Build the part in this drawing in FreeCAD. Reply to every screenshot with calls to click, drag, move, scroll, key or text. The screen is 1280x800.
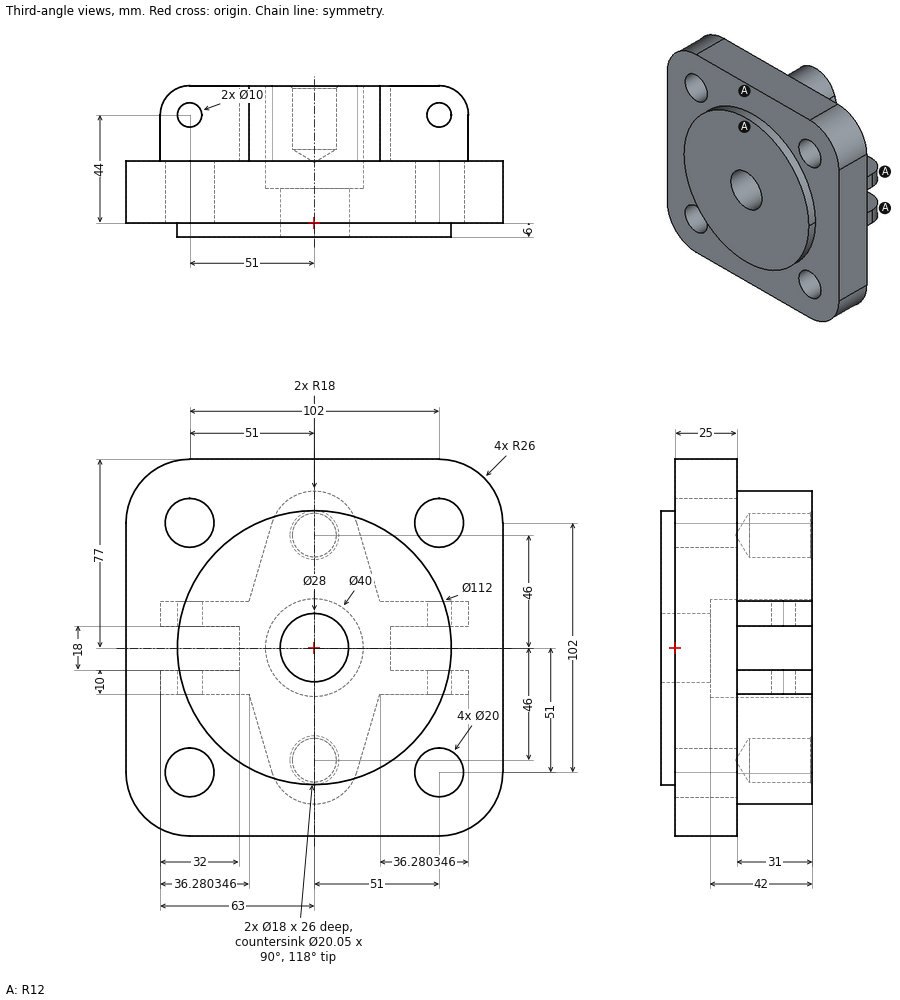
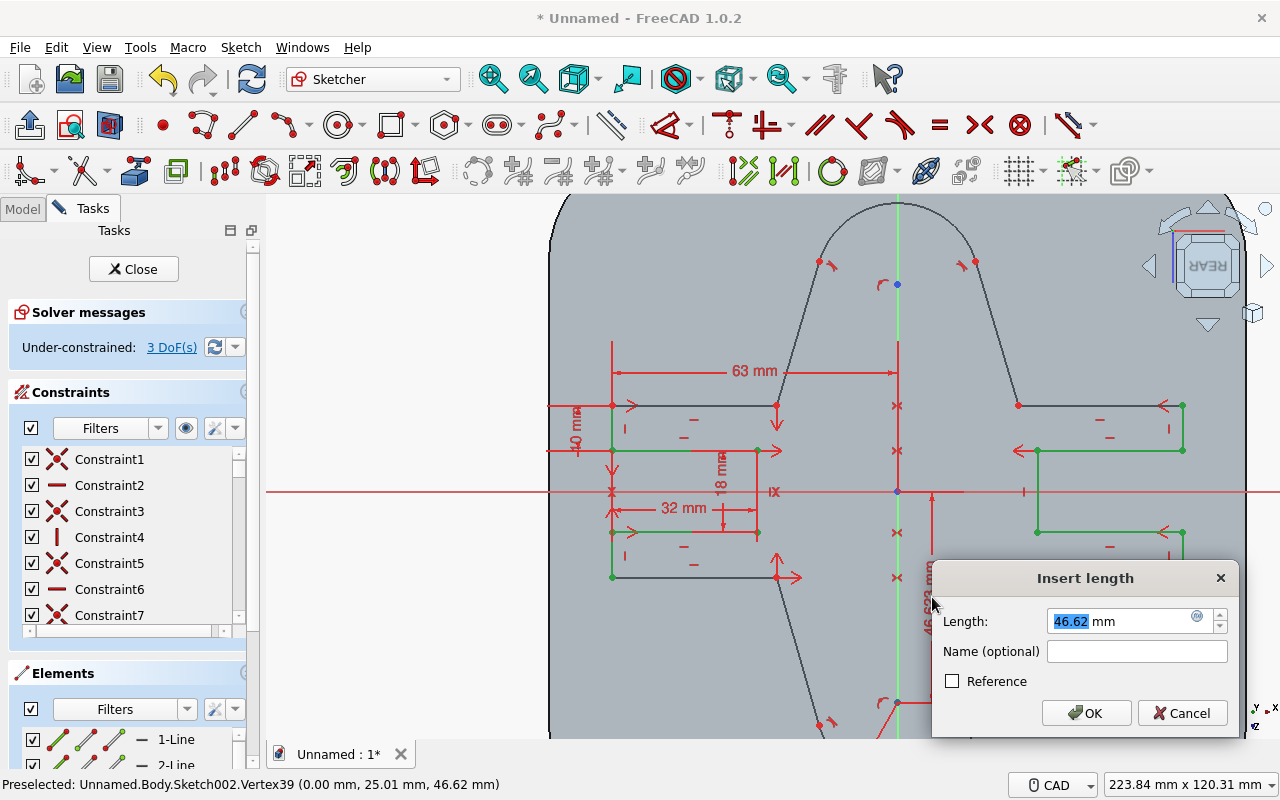
text(46)
key(Return)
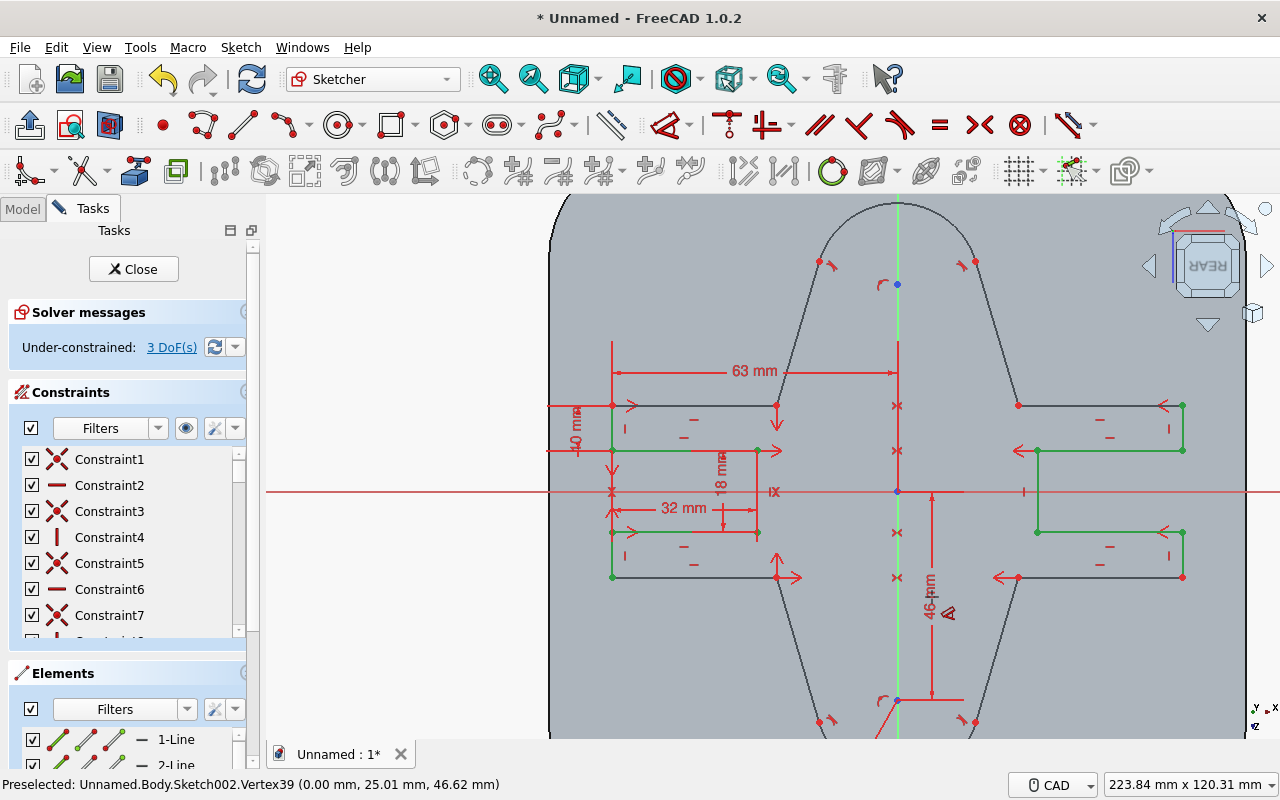
click(898, 285)
click(932, 388)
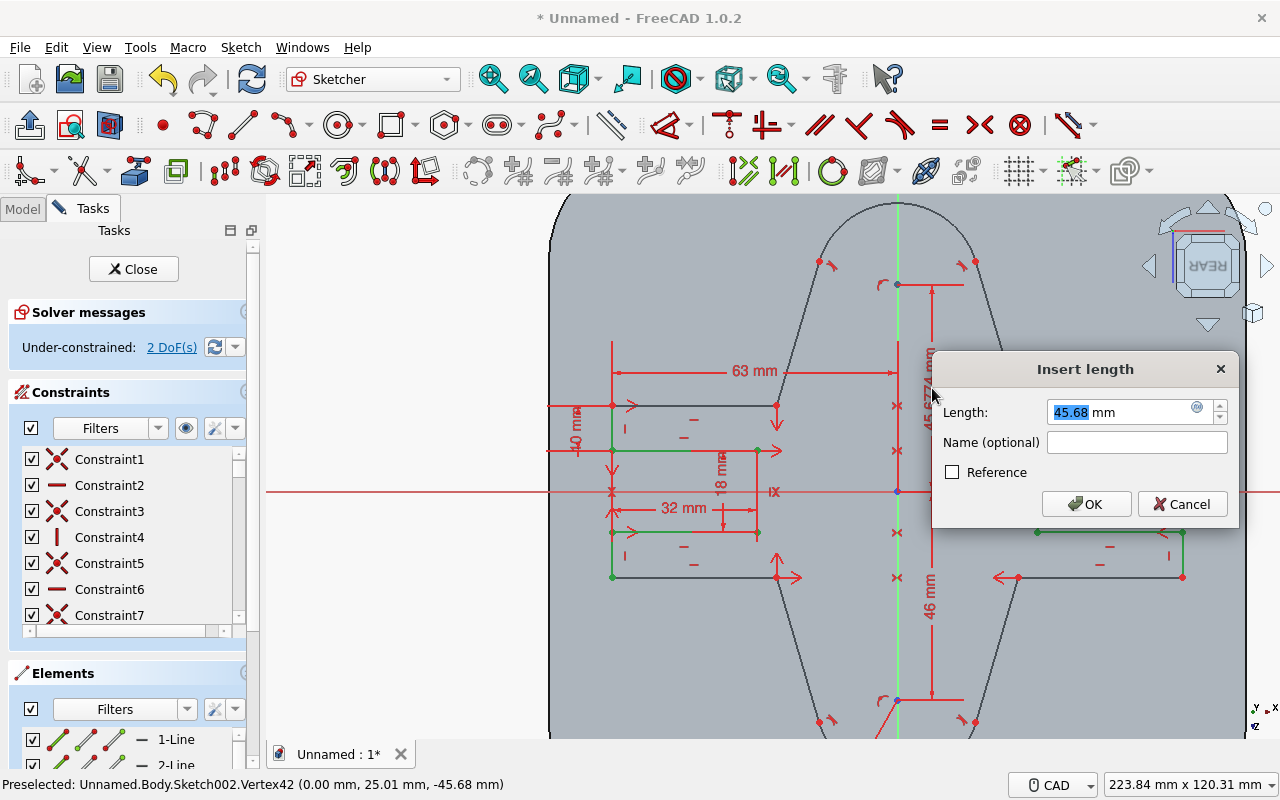
text(46)
key(Return)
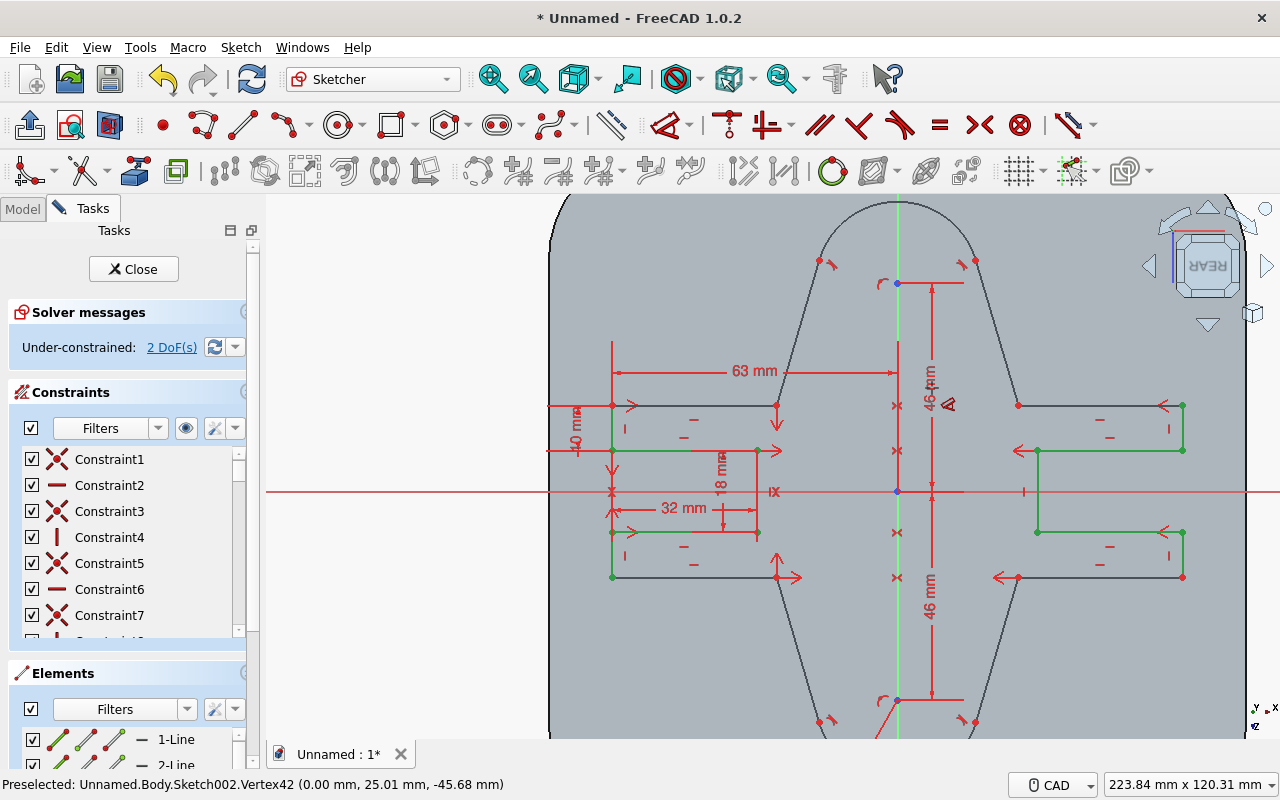
click(727, 406)
click(657, 372)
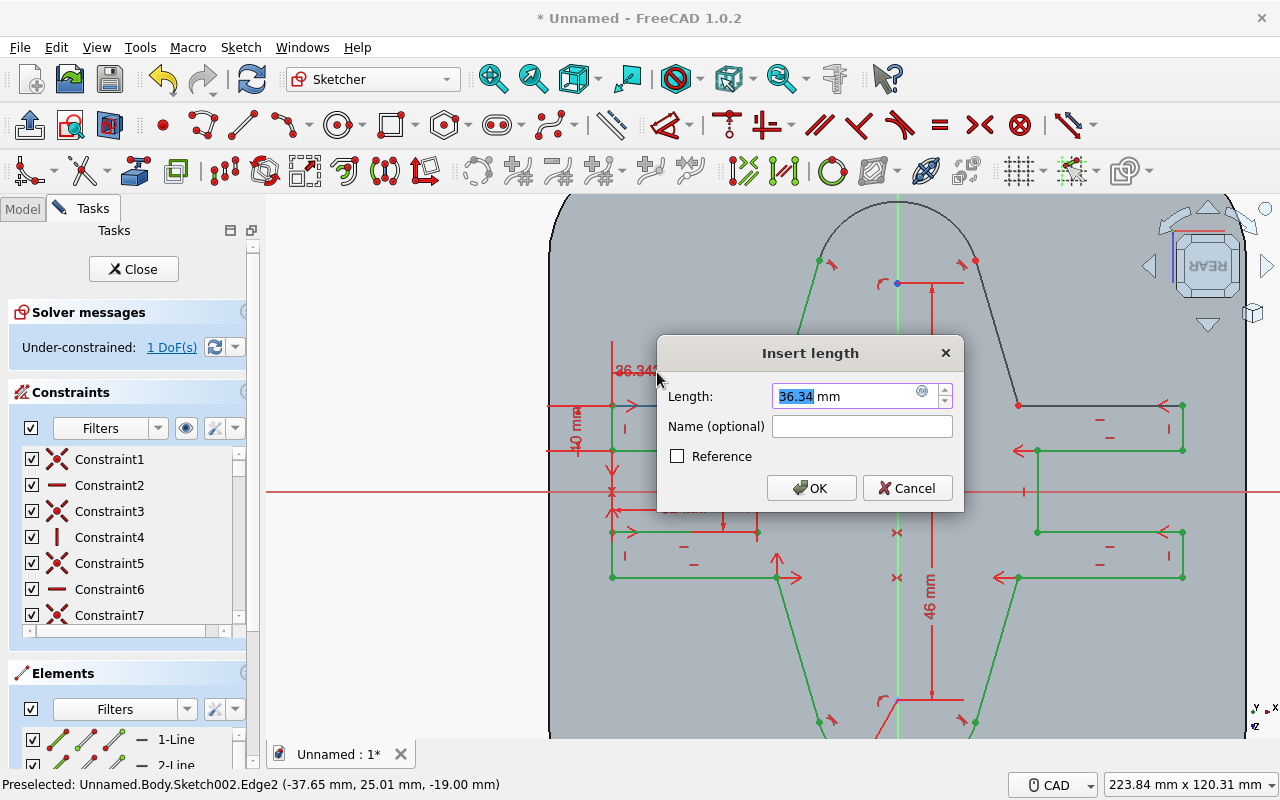
text(36.280346)
key(Return)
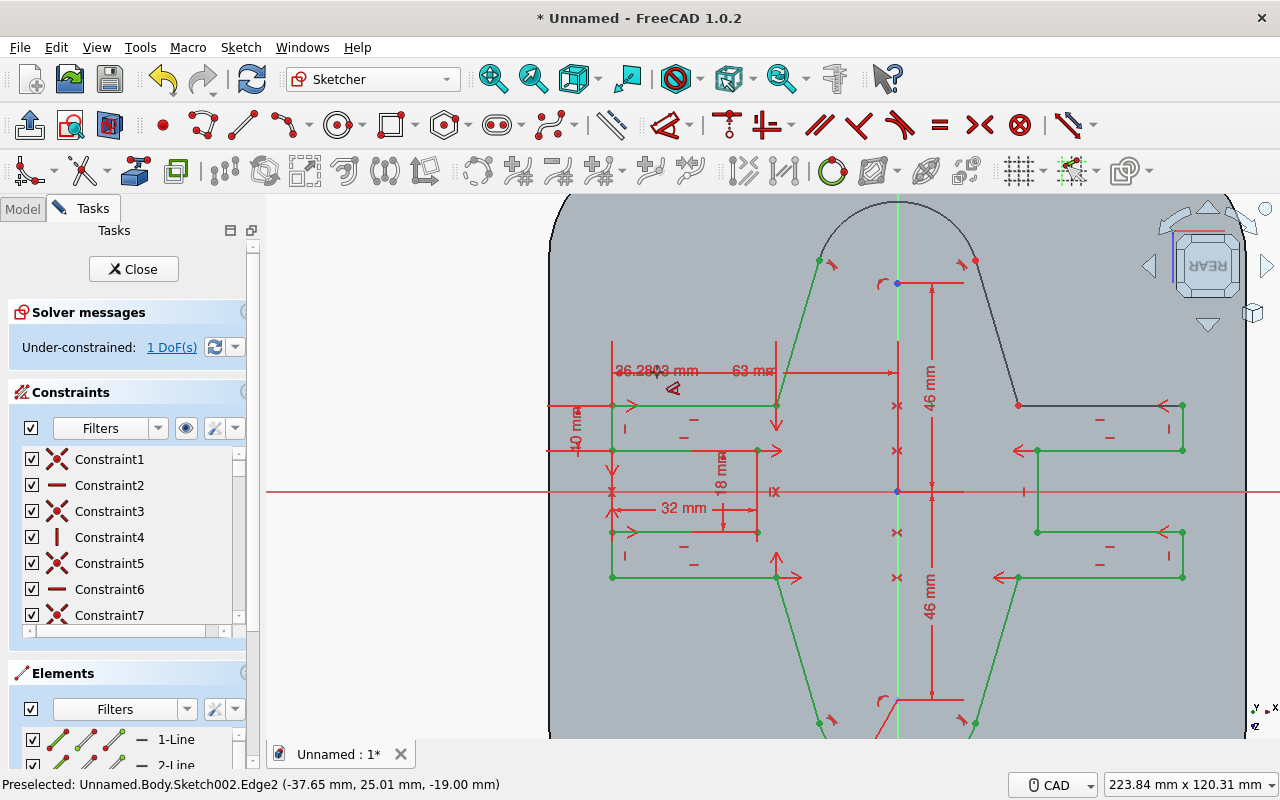
click(1068, 406)
click(1067, 372)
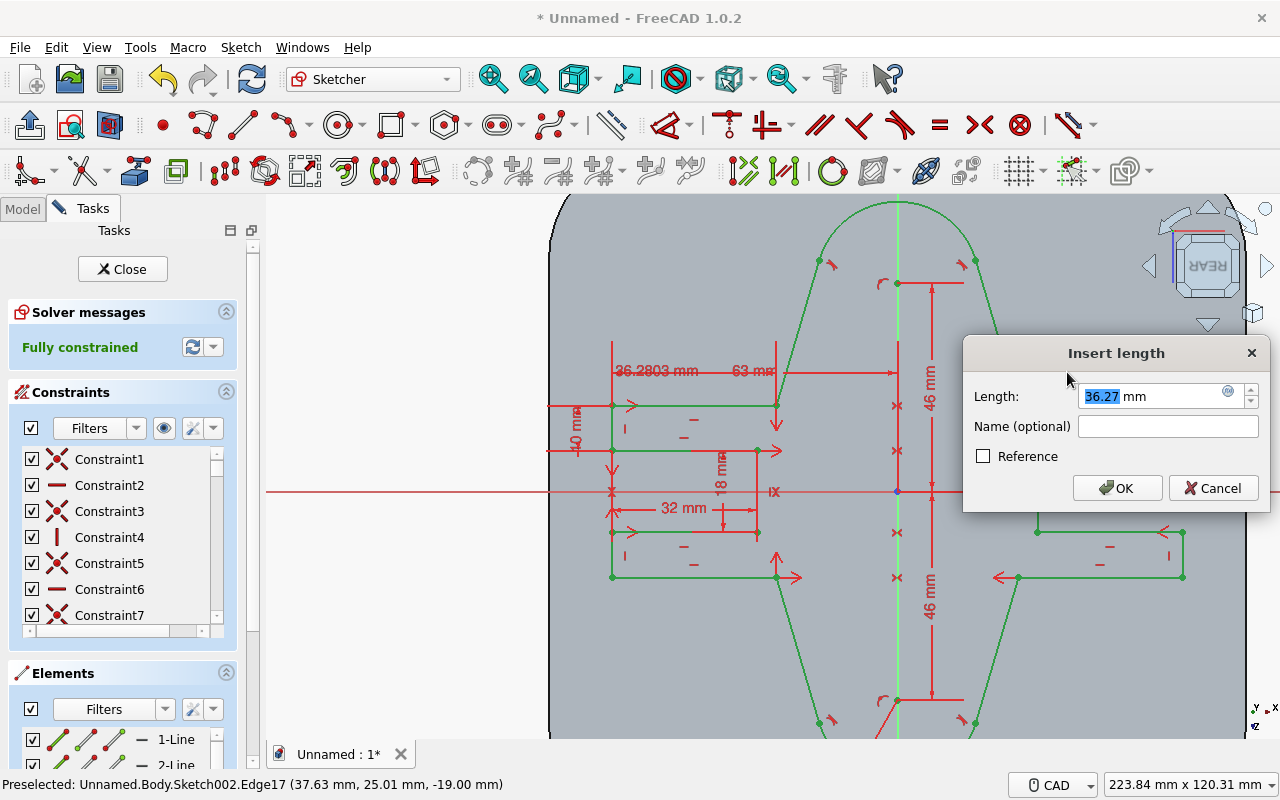
text(36.280346)
key(Return)
key(Escape)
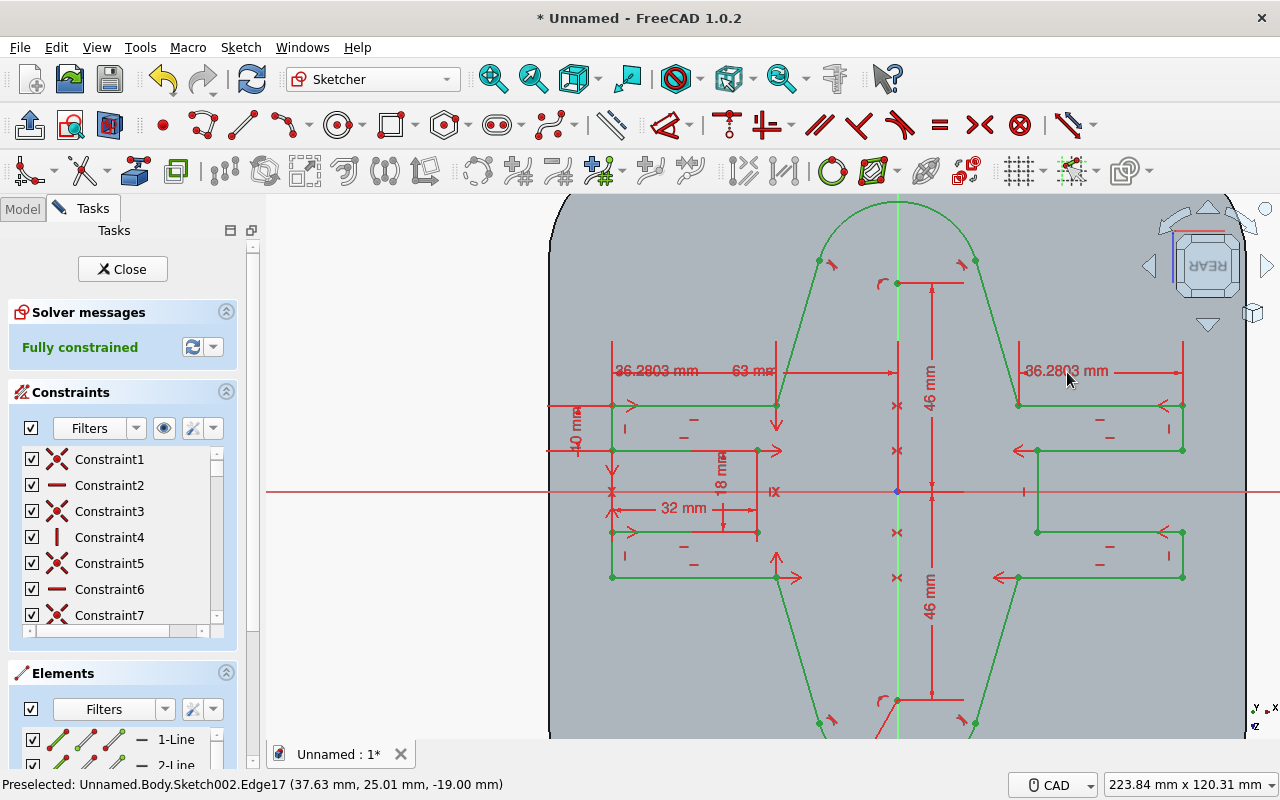
click(123, 269)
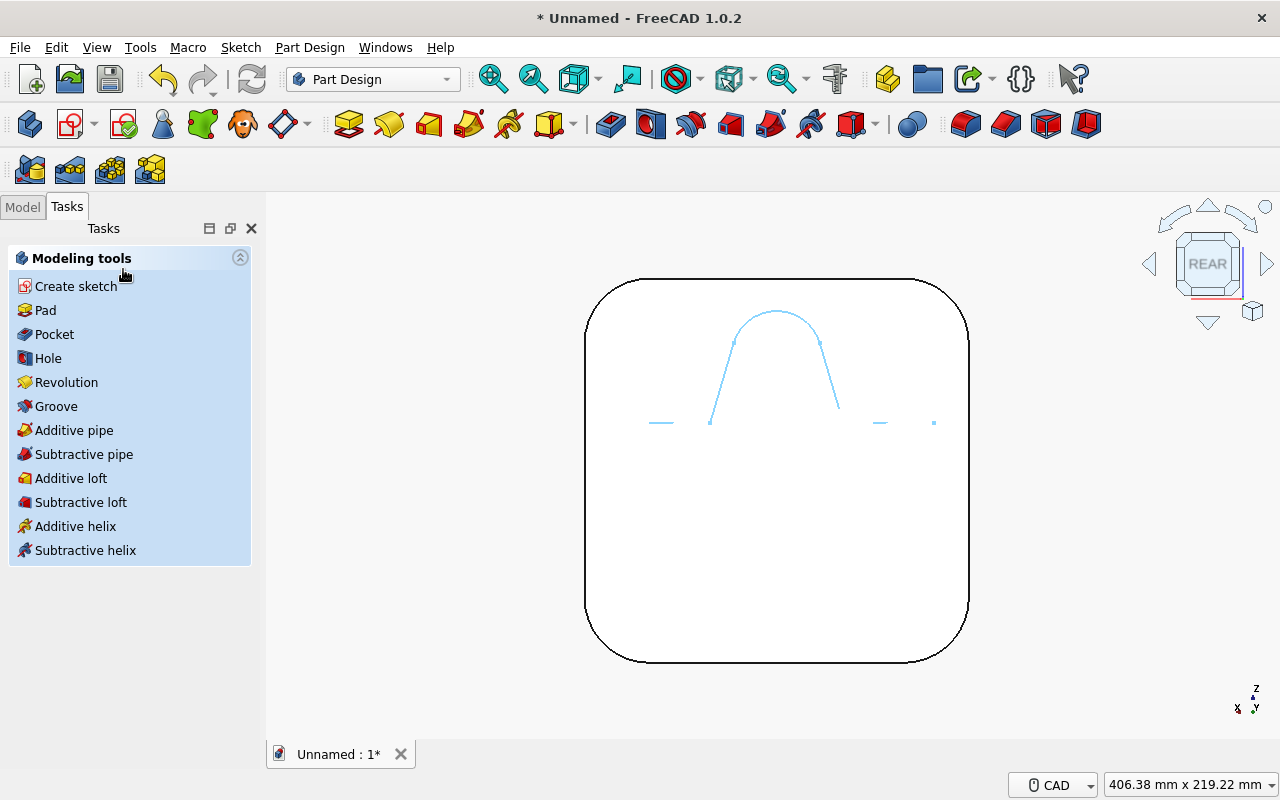
click(350, 124)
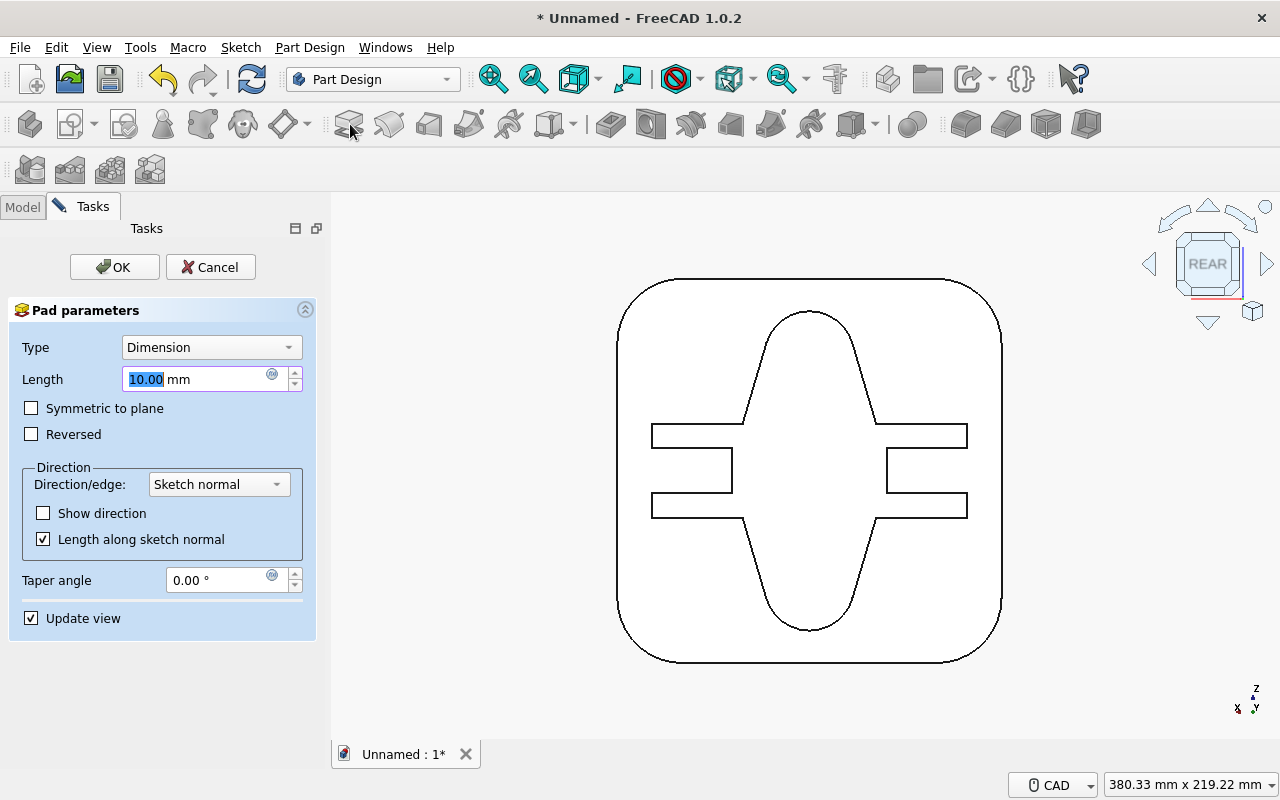
text(31)
key(Tab)